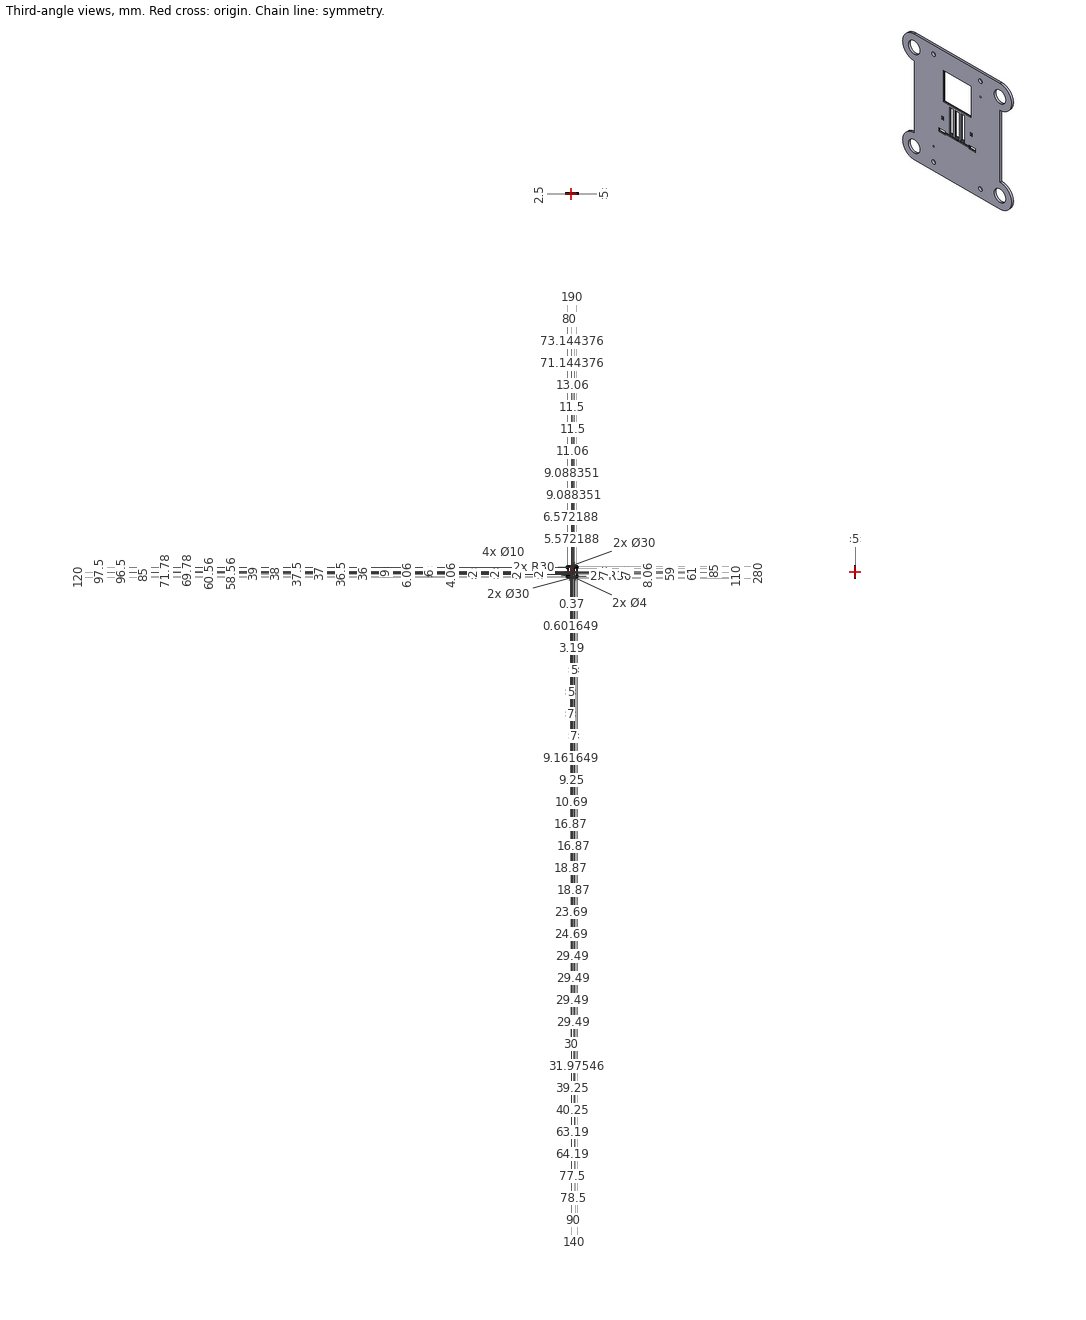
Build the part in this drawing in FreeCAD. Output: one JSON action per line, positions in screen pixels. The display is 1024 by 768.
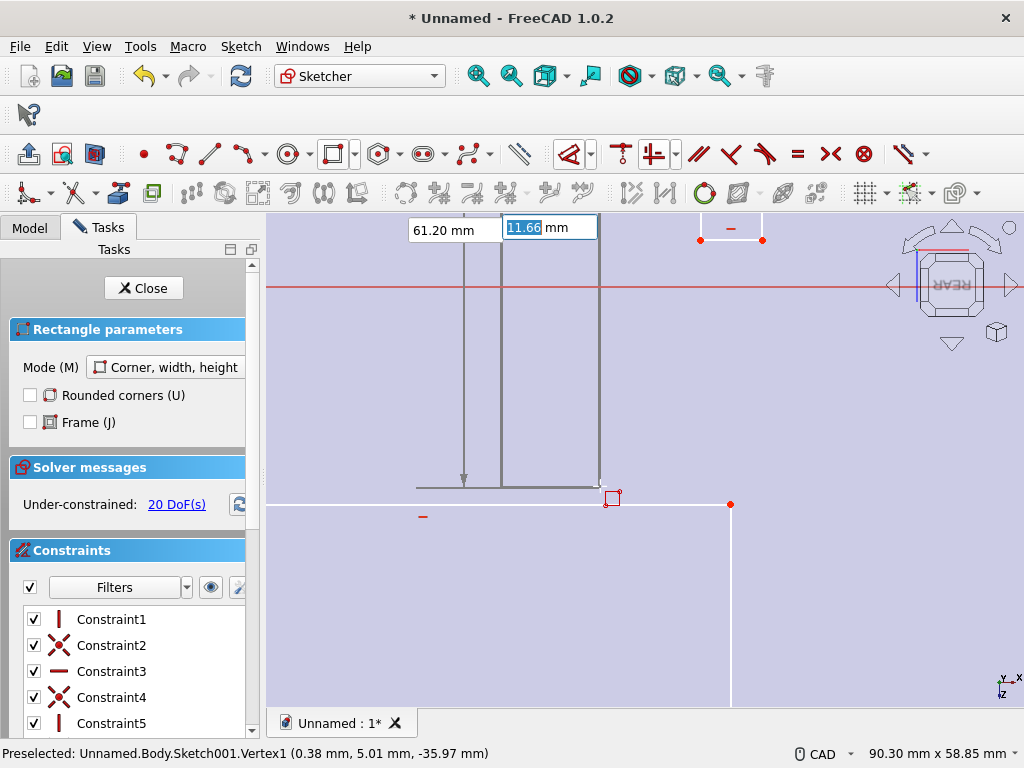
{"action": "left_click", "coordinate": [598, 484]}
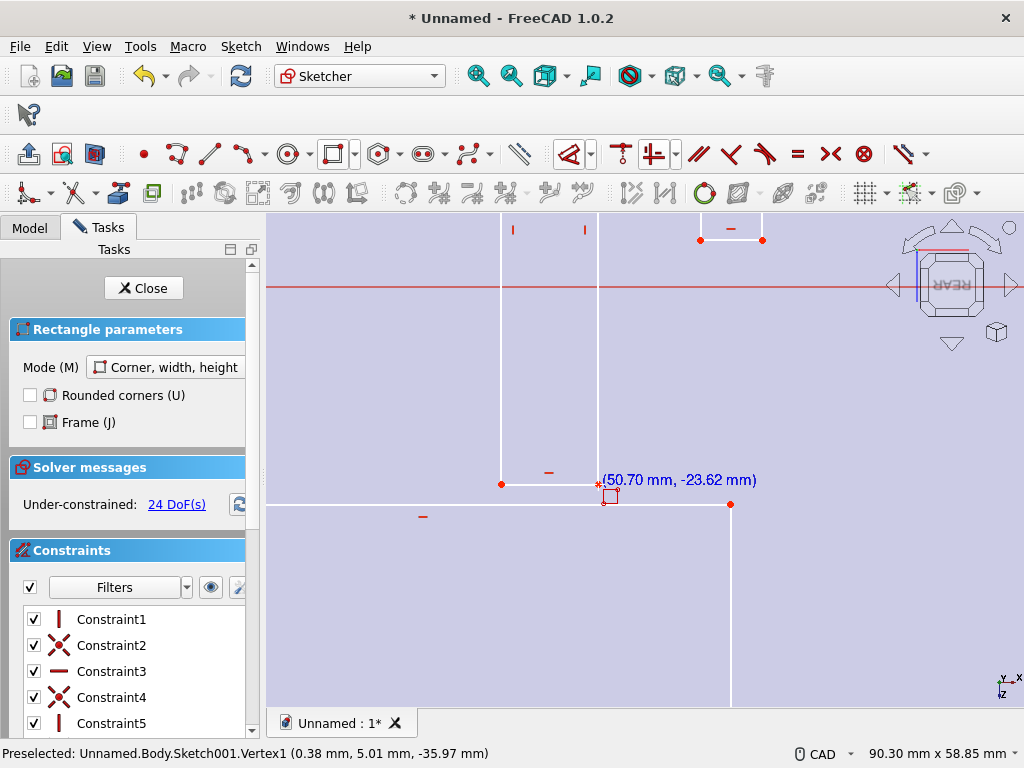
{"action": "scroll", "coordinate": [626, 446], "scroll_direction": "down", "scroll_amount": 7}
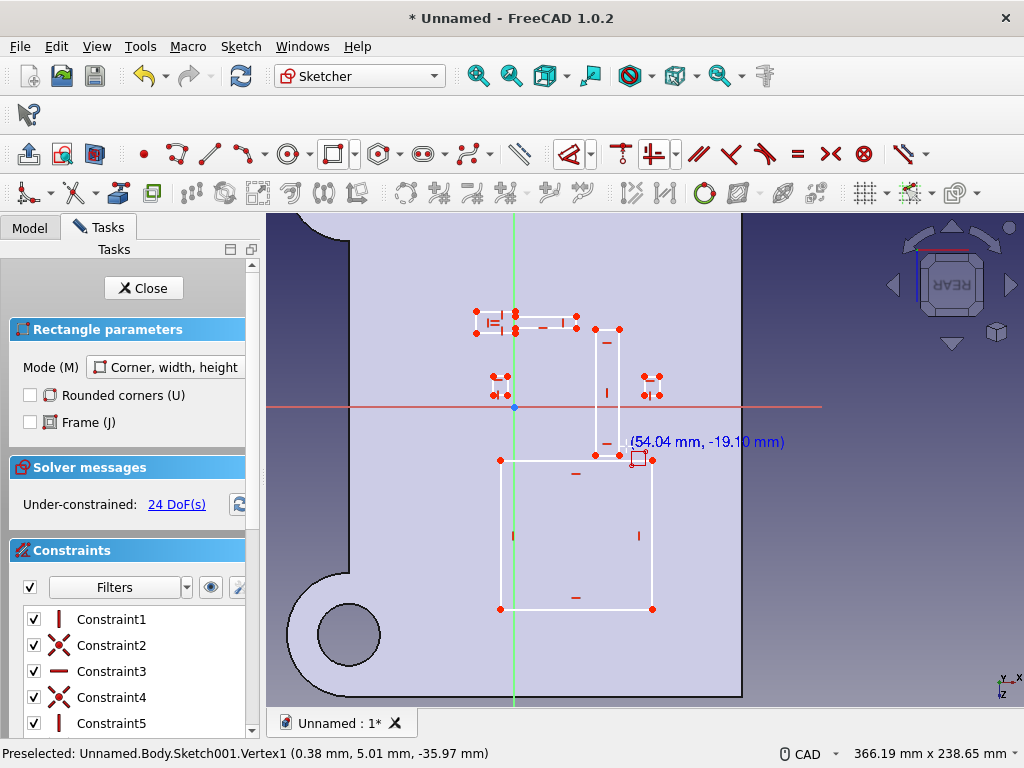
{"action": "scroll", "coordinate": [564, 329], "scroll_direction": "up", "scroll_amount": 14}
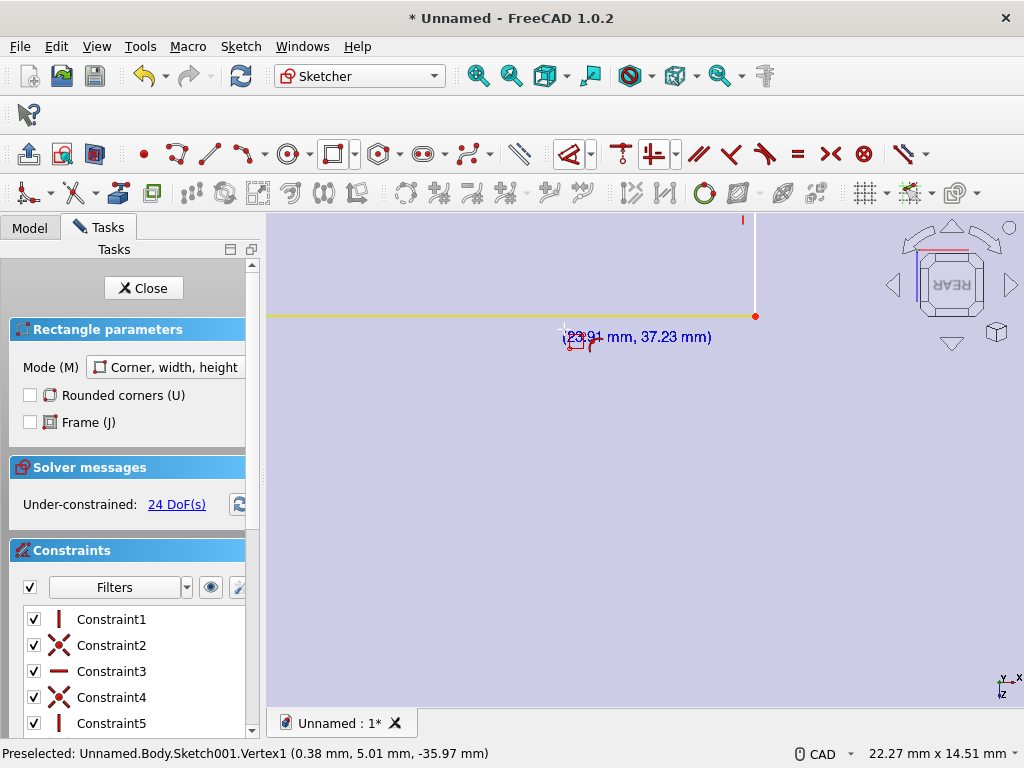
{"action": "left_click", "coordinate": [550, 333]}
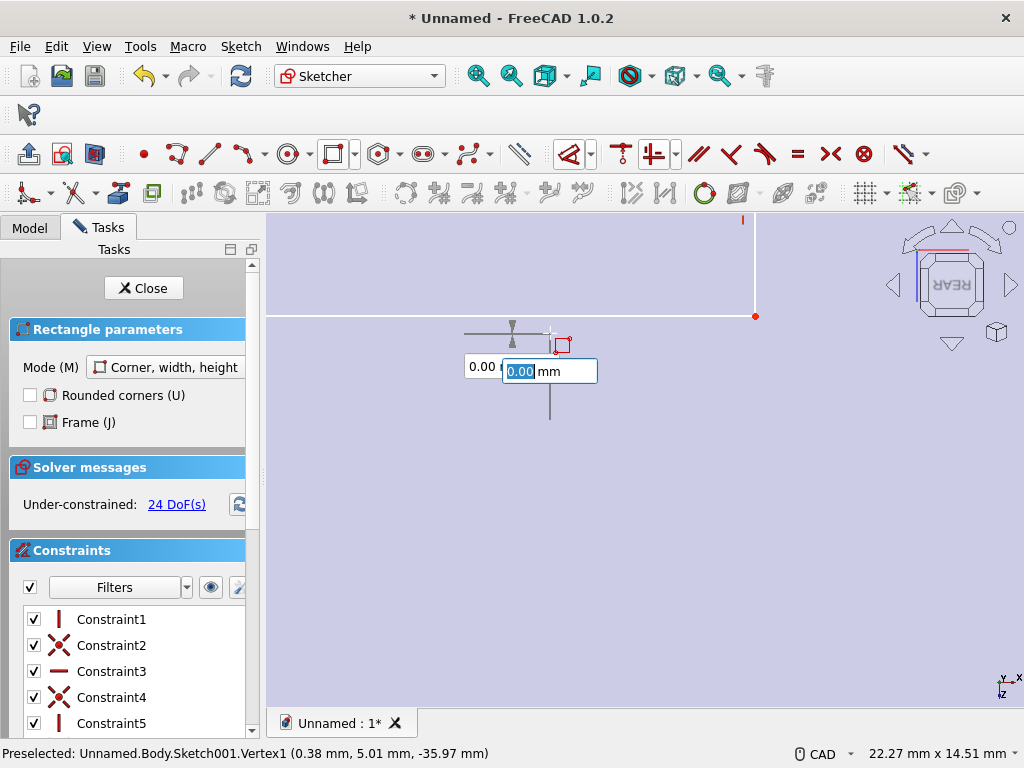
{"action": "scroll", "coordinate": [564, 329], "scroll_direction": "down", "scroll_amount": 14}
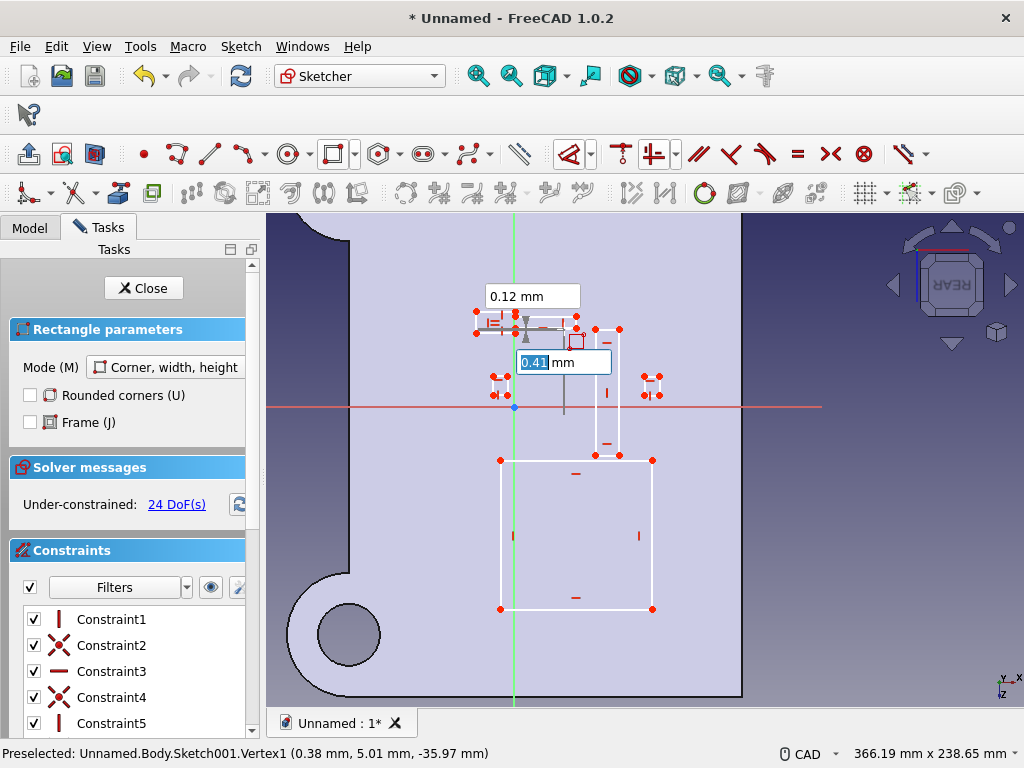
{"action": "scroll", "coordinate": [591, 455], "scroll_direction": "up", "scroll_amount": 6}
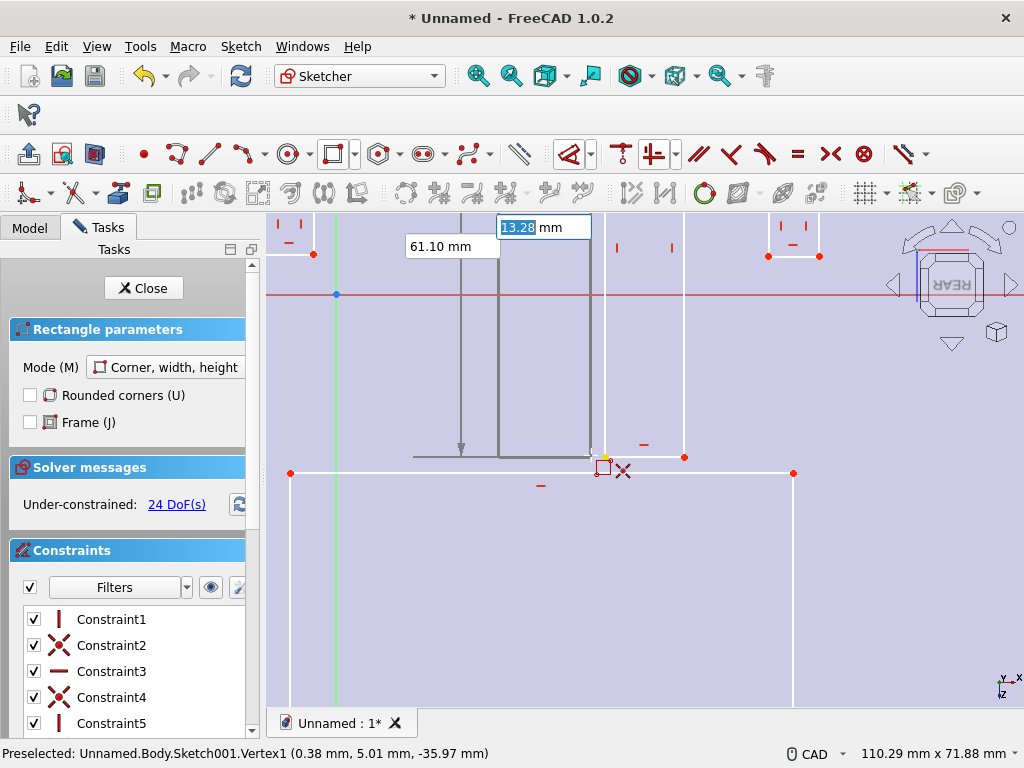
{"action": "left_click", "coordinate": [589, 453]}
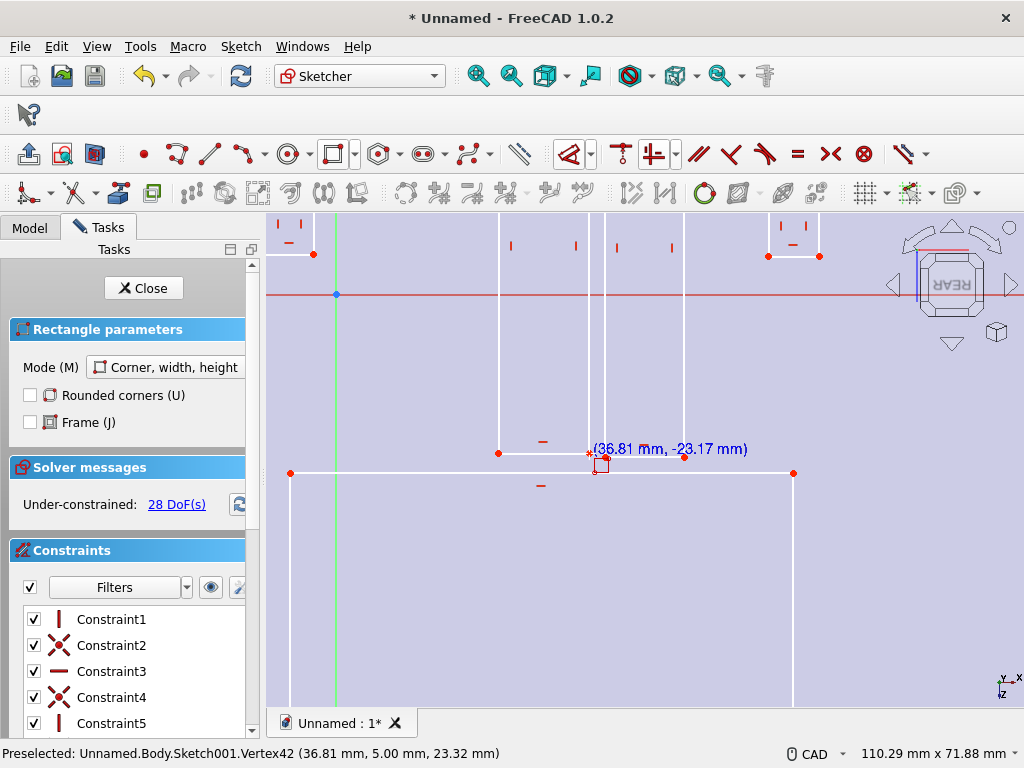
{"action": "scroll", "coordinate": [591, 455], "scroll_direction": "down", "scroll_amount": 6}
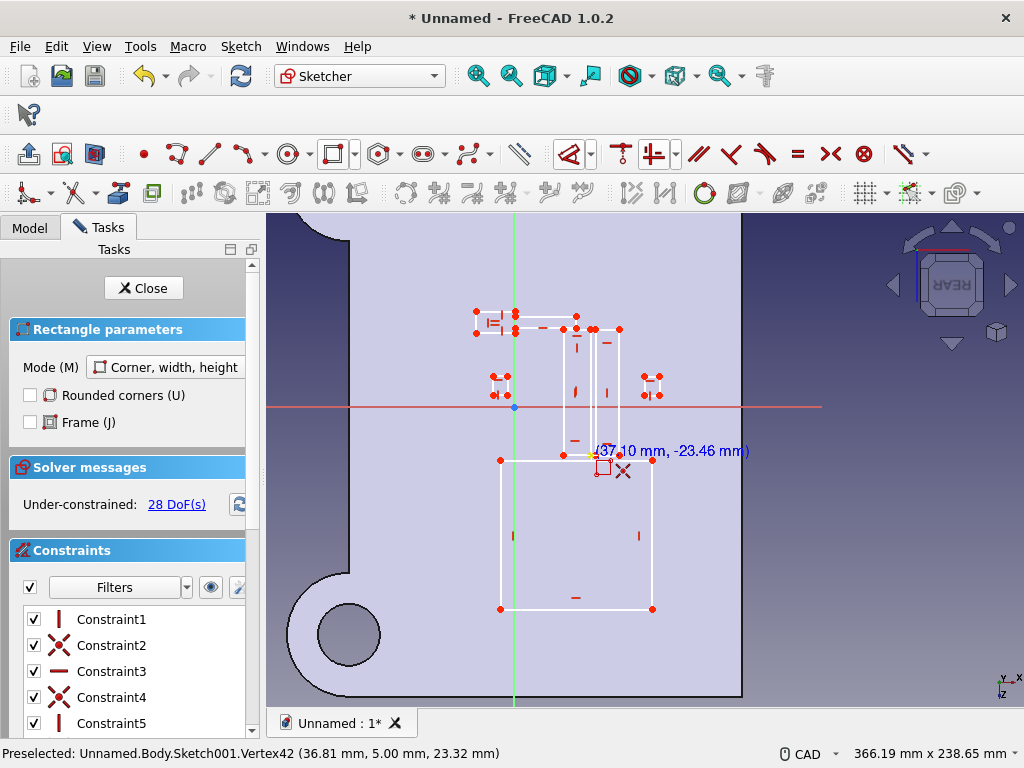
{"action": "scroll", "coordinate": [534, 329], "scroll_direction": "up", "scroll_amount": 14}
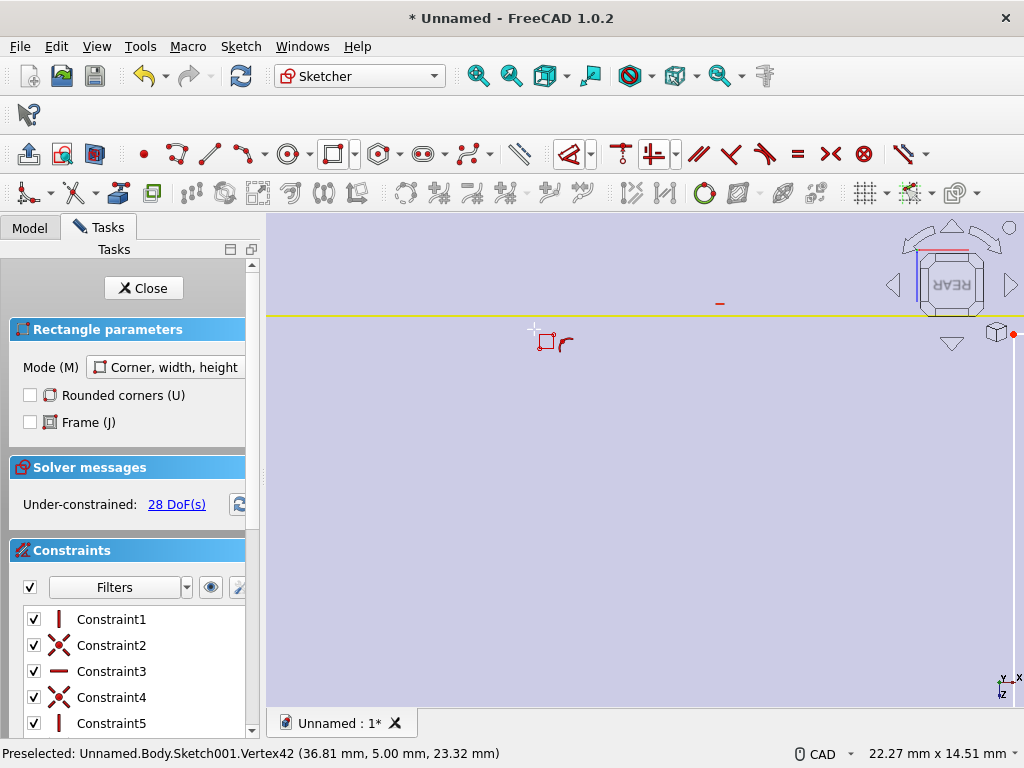
{"action": "left_click", "coordinate": [523, 333]}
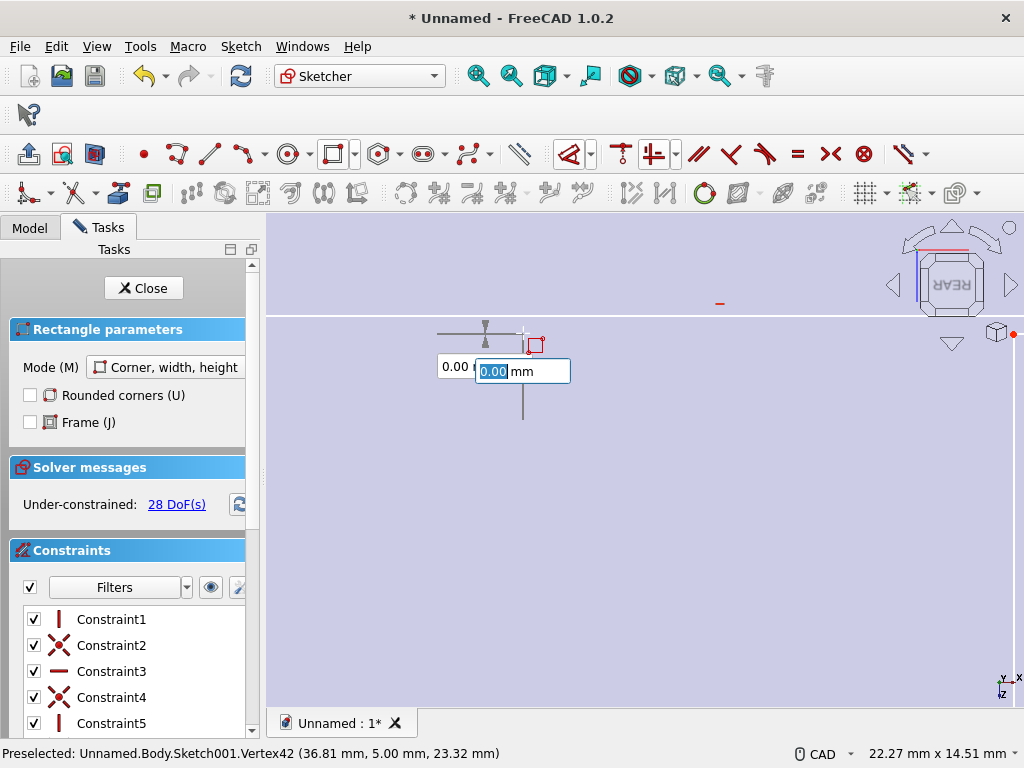
{"action": "scroll", "coordinate": [534, 329], "scroll_direction": "down", "scroll_amount": 14}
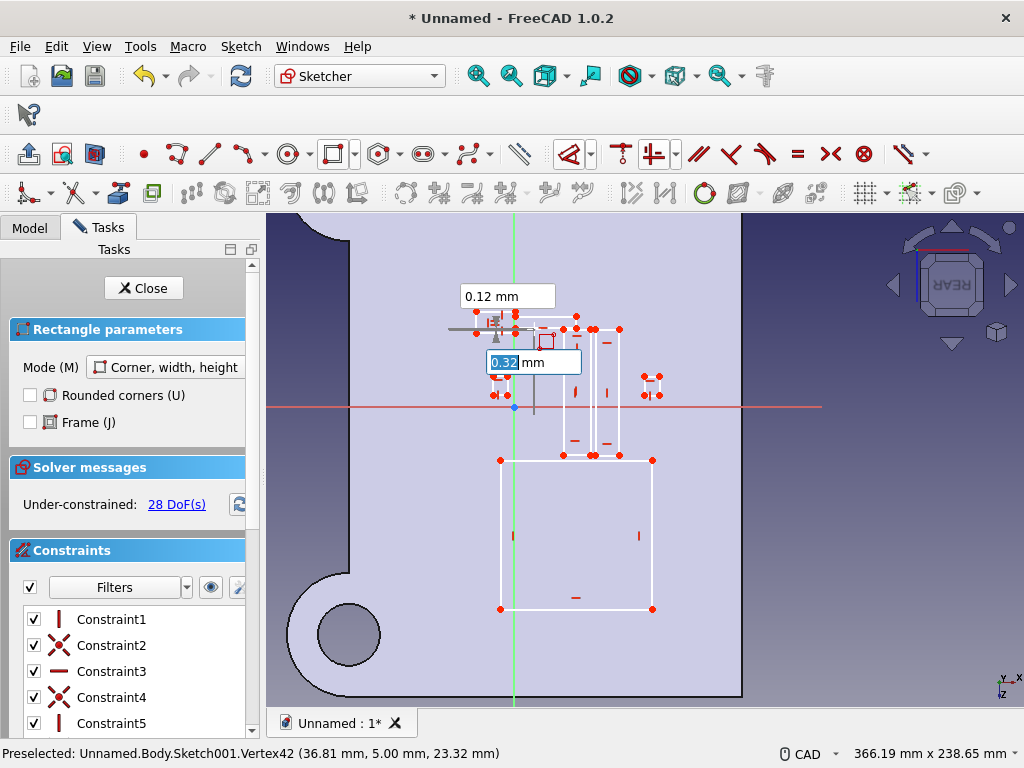
{"action": "scroll", "coordinate": [557, 456], "scroll_direction": "up", "scroll_amount": 7}